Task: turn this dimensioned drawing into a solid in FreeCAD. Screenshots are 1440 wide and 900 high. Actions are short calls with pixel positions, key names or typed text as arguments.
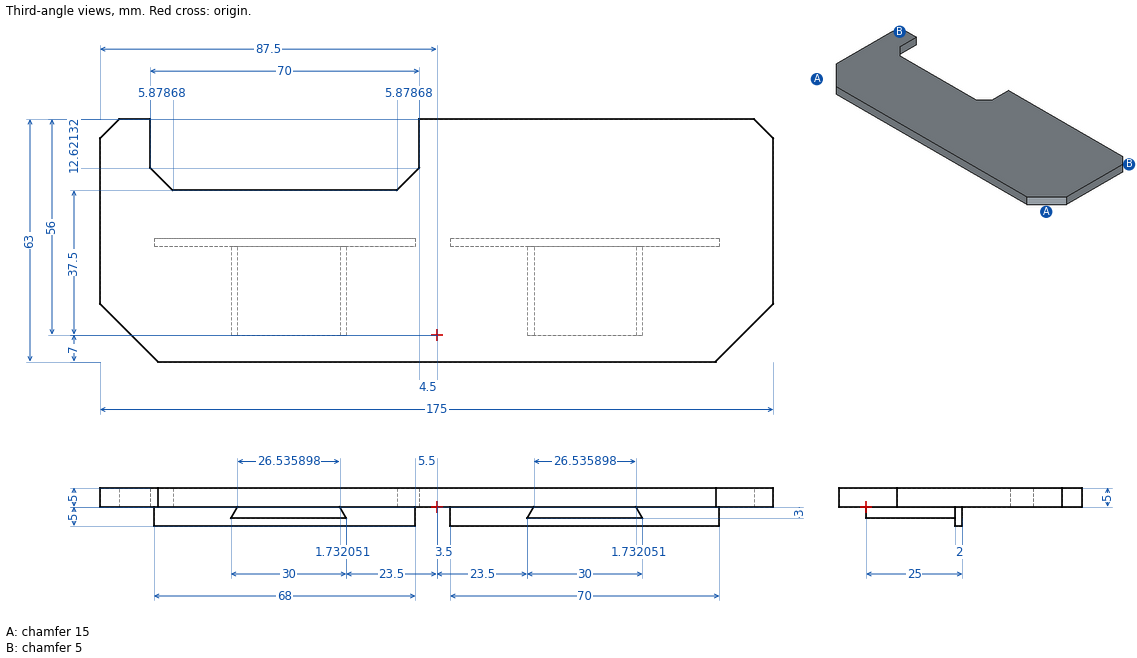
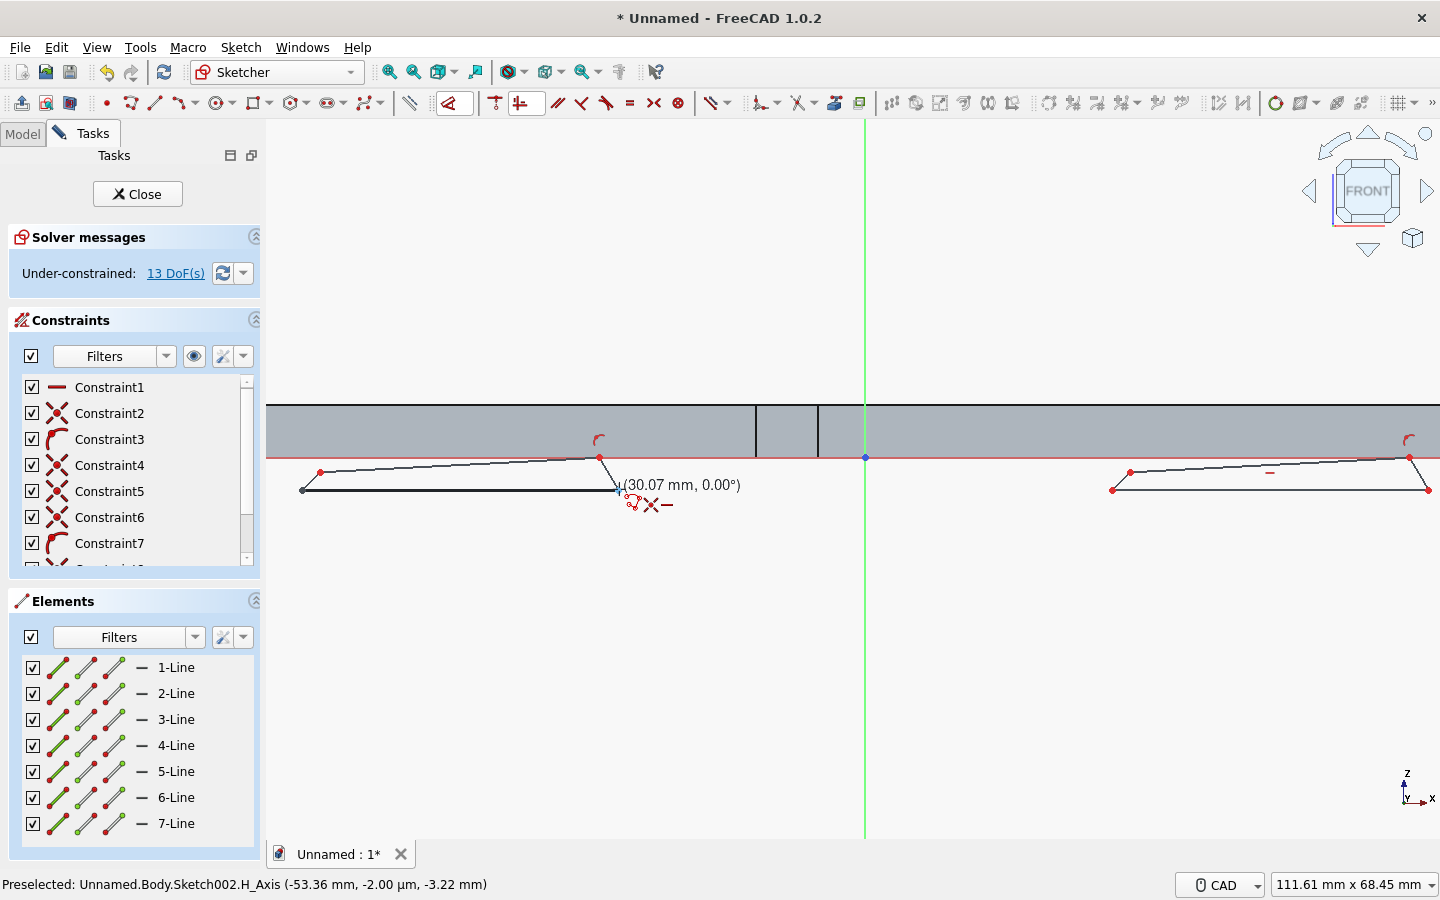
click(619, 490)
key(Escape)
key(Escape)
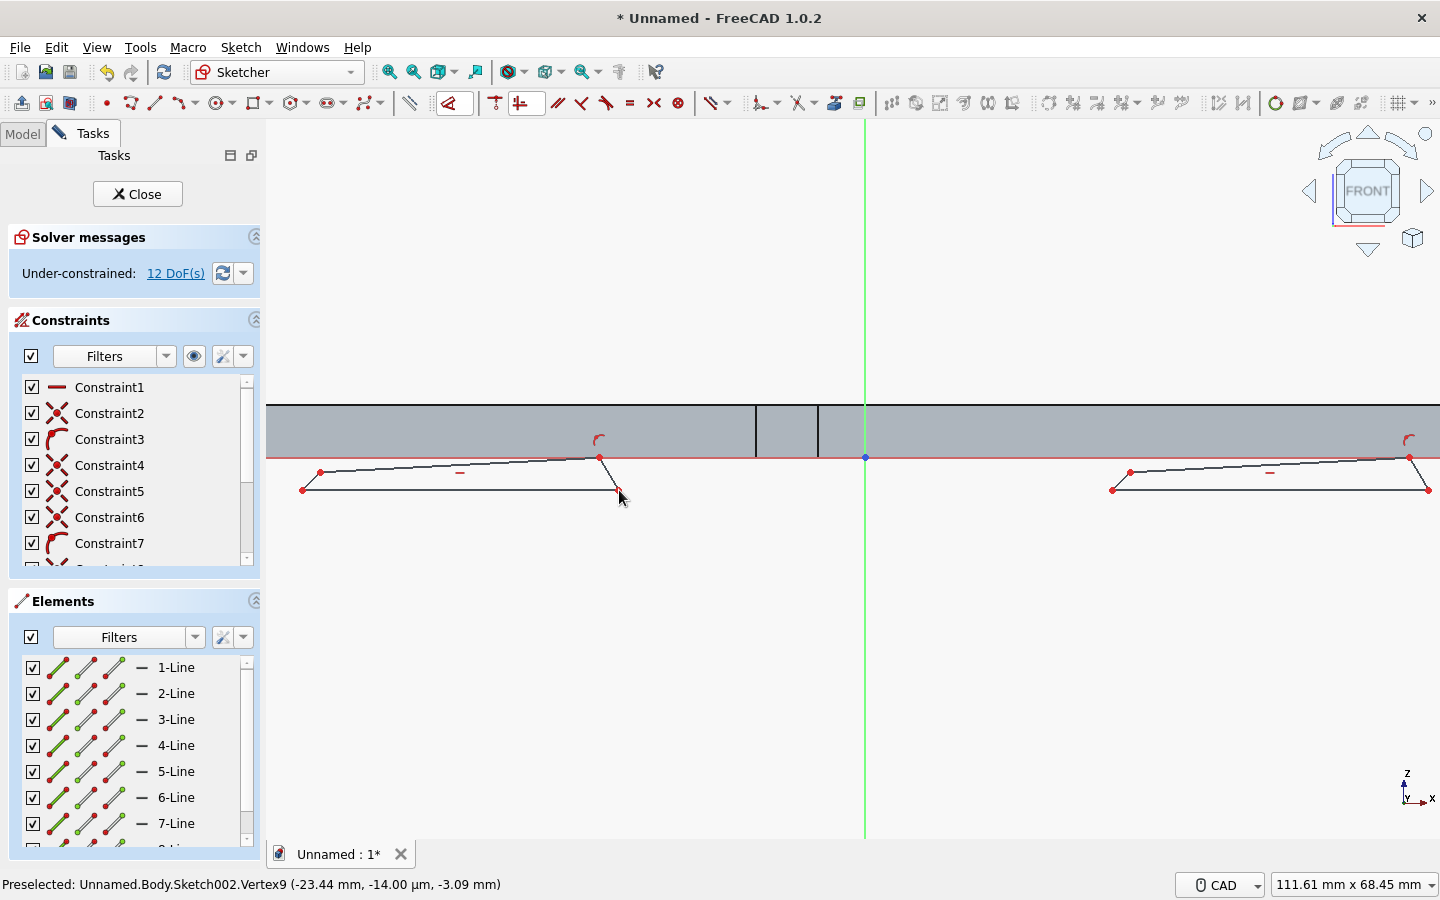
scroll(1214, 468, up, 2)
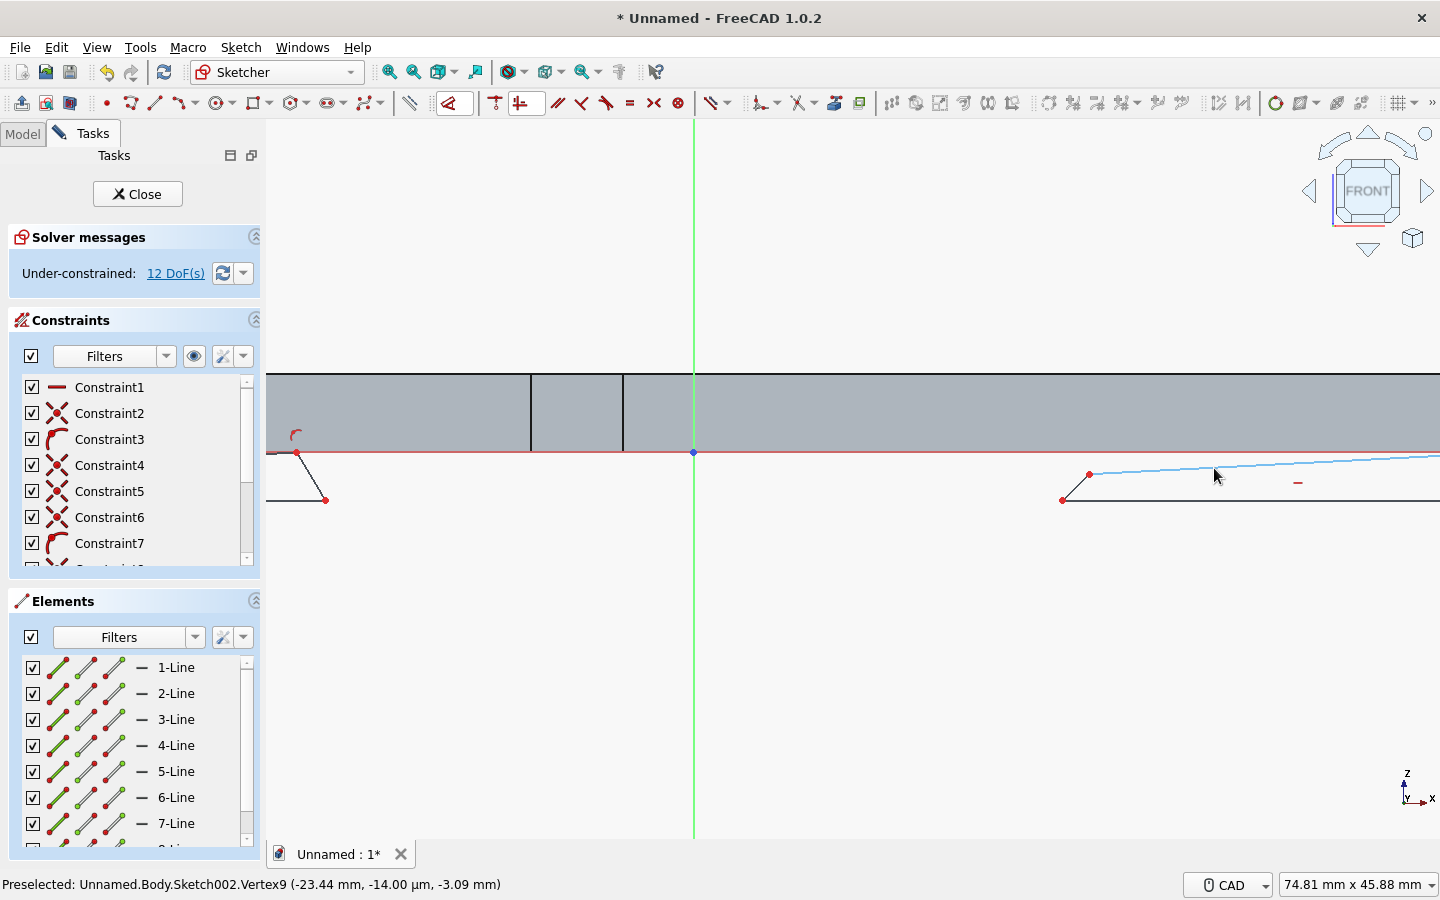
click(1214, 468)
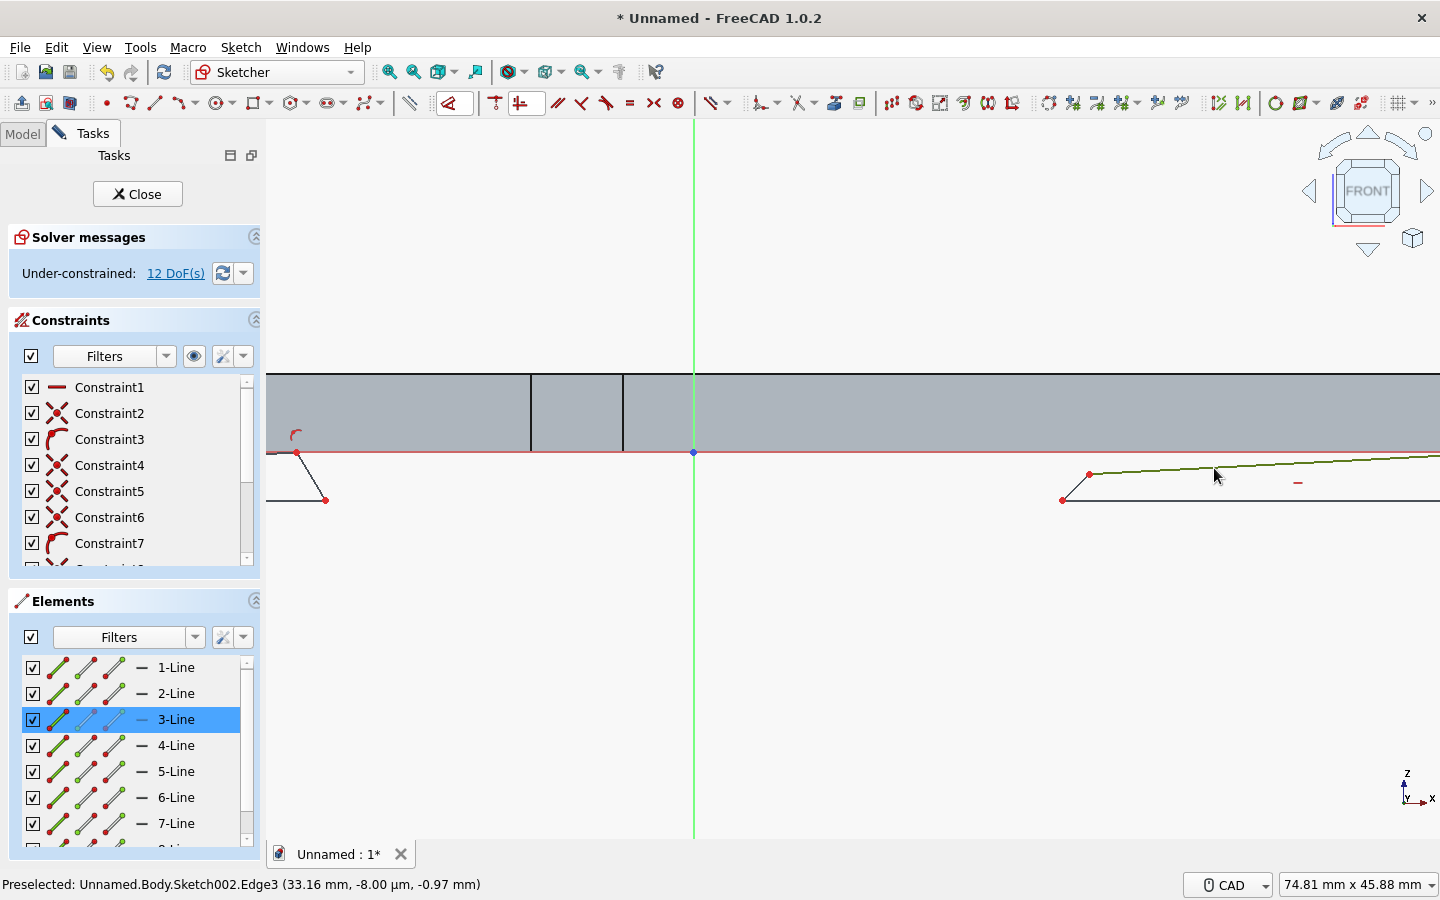
key(h)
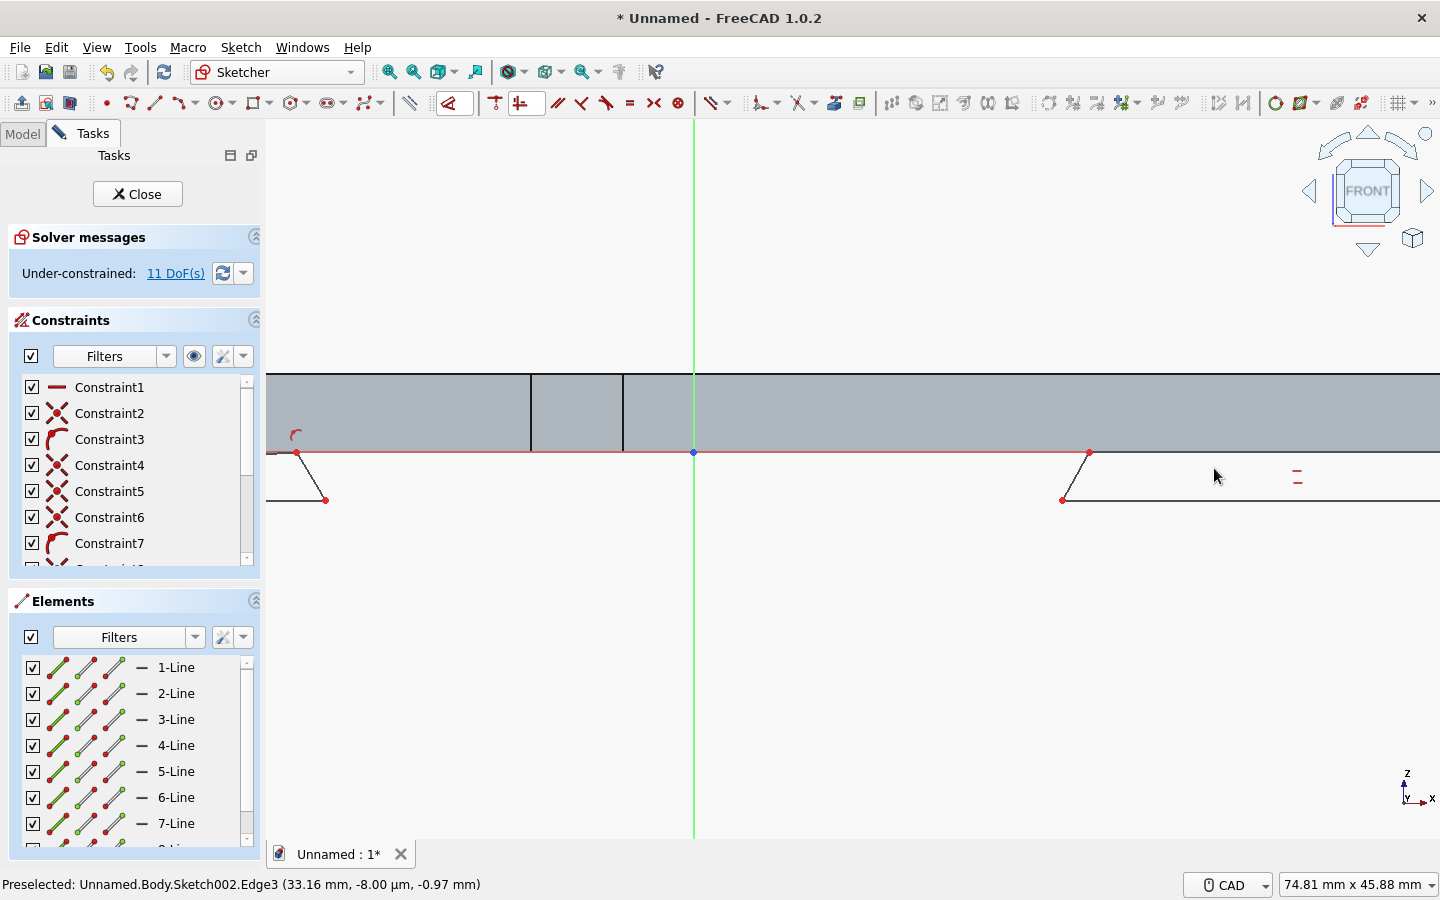
scroll(859, 481, down, 4)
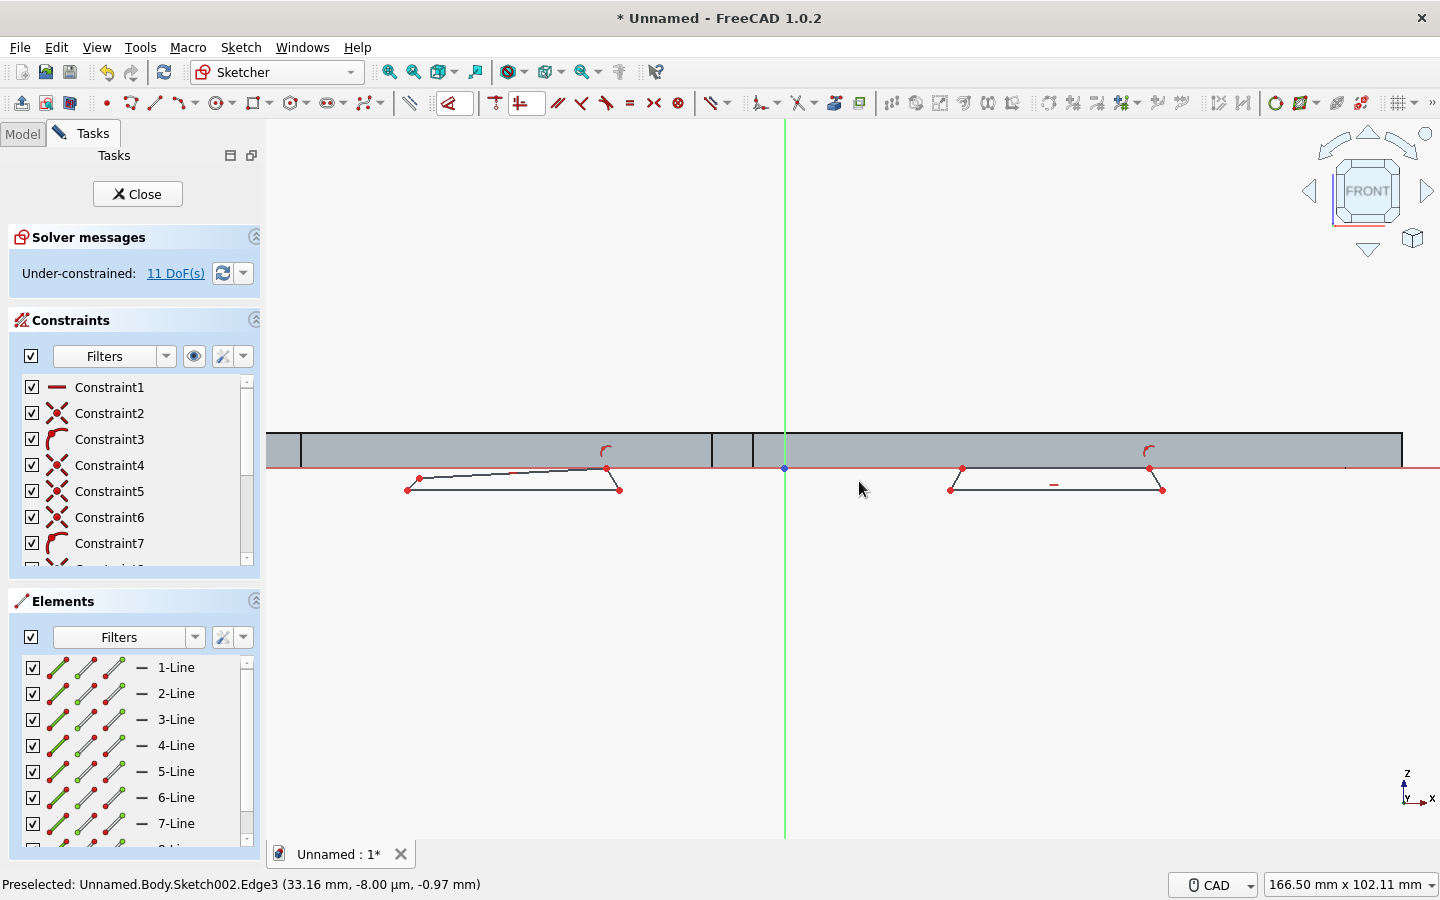
scroll(476, 475, up, 4)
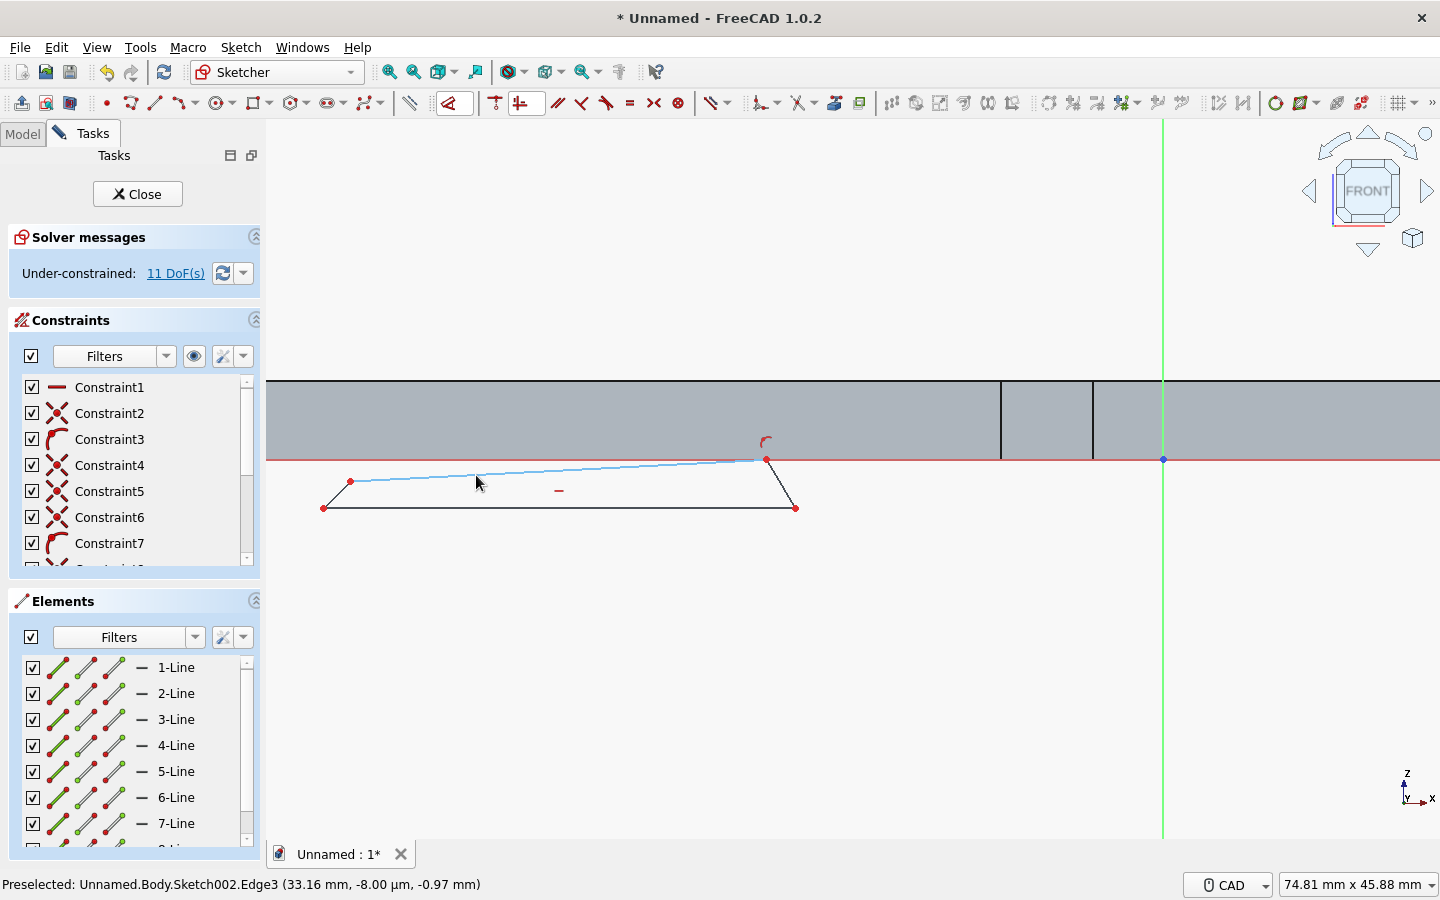
click(475, 475)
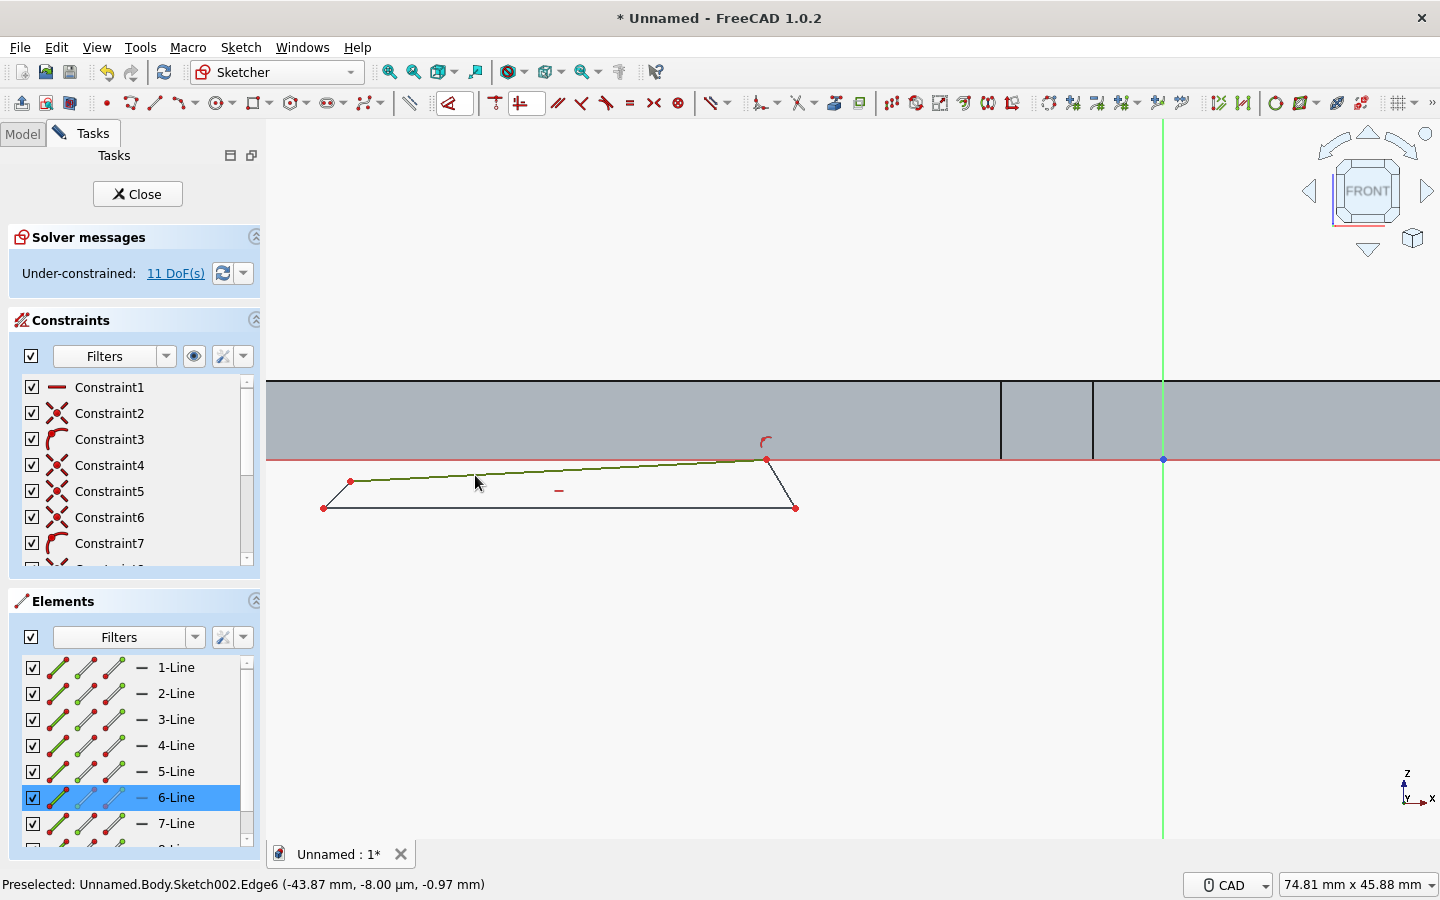
key(h)